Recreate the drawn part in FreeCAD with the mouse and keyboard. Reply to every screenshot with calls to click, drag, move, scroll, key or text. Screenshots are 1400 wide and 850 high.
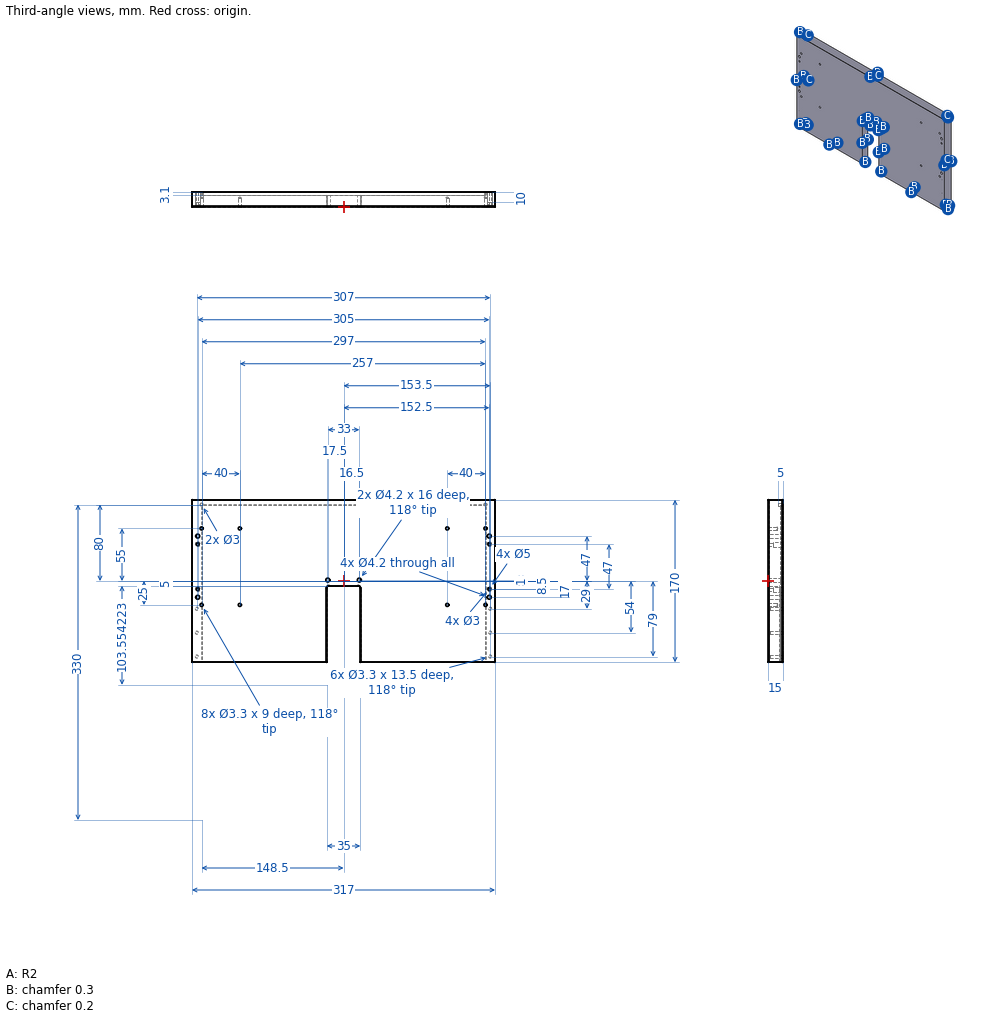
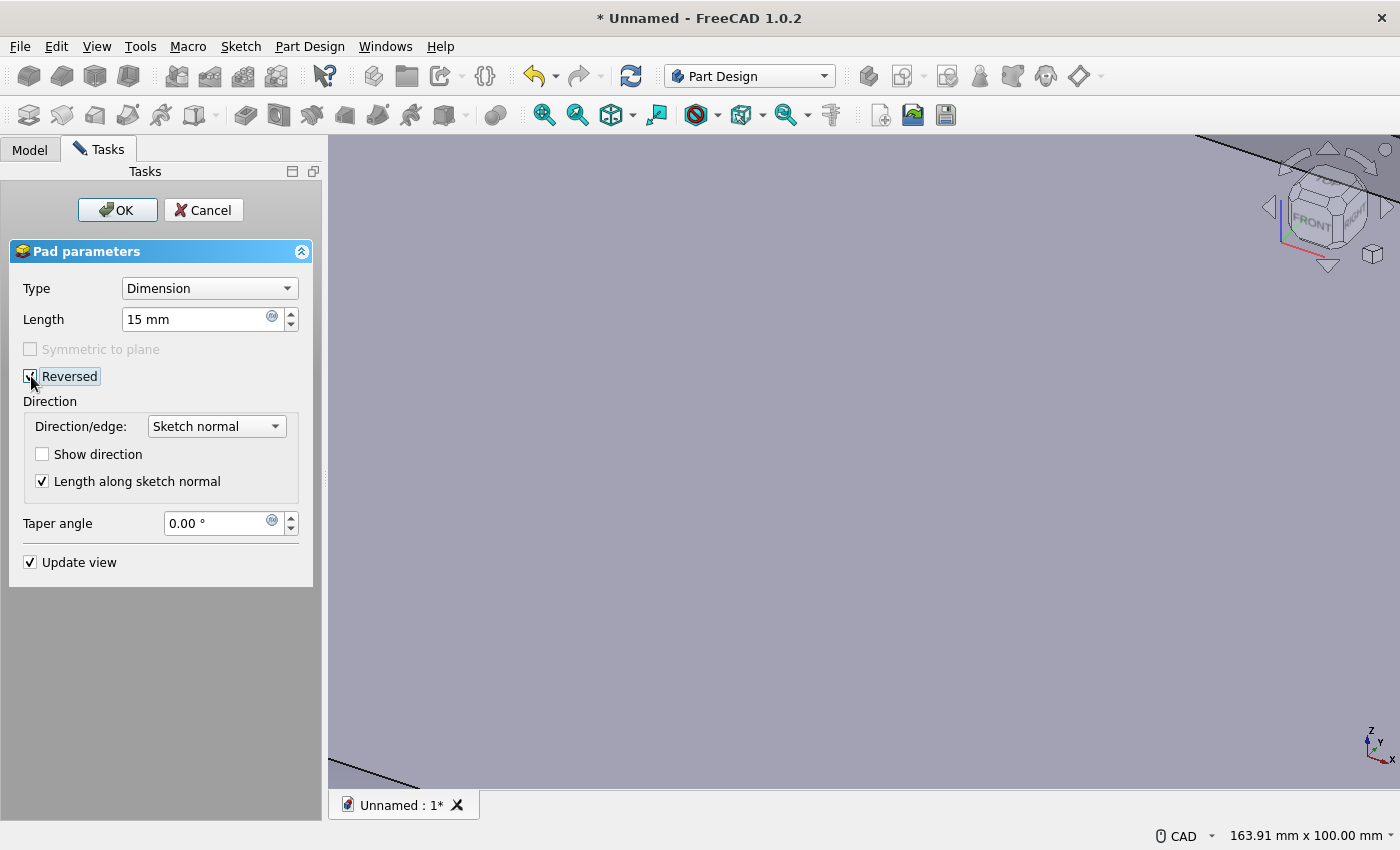
click(118, 210)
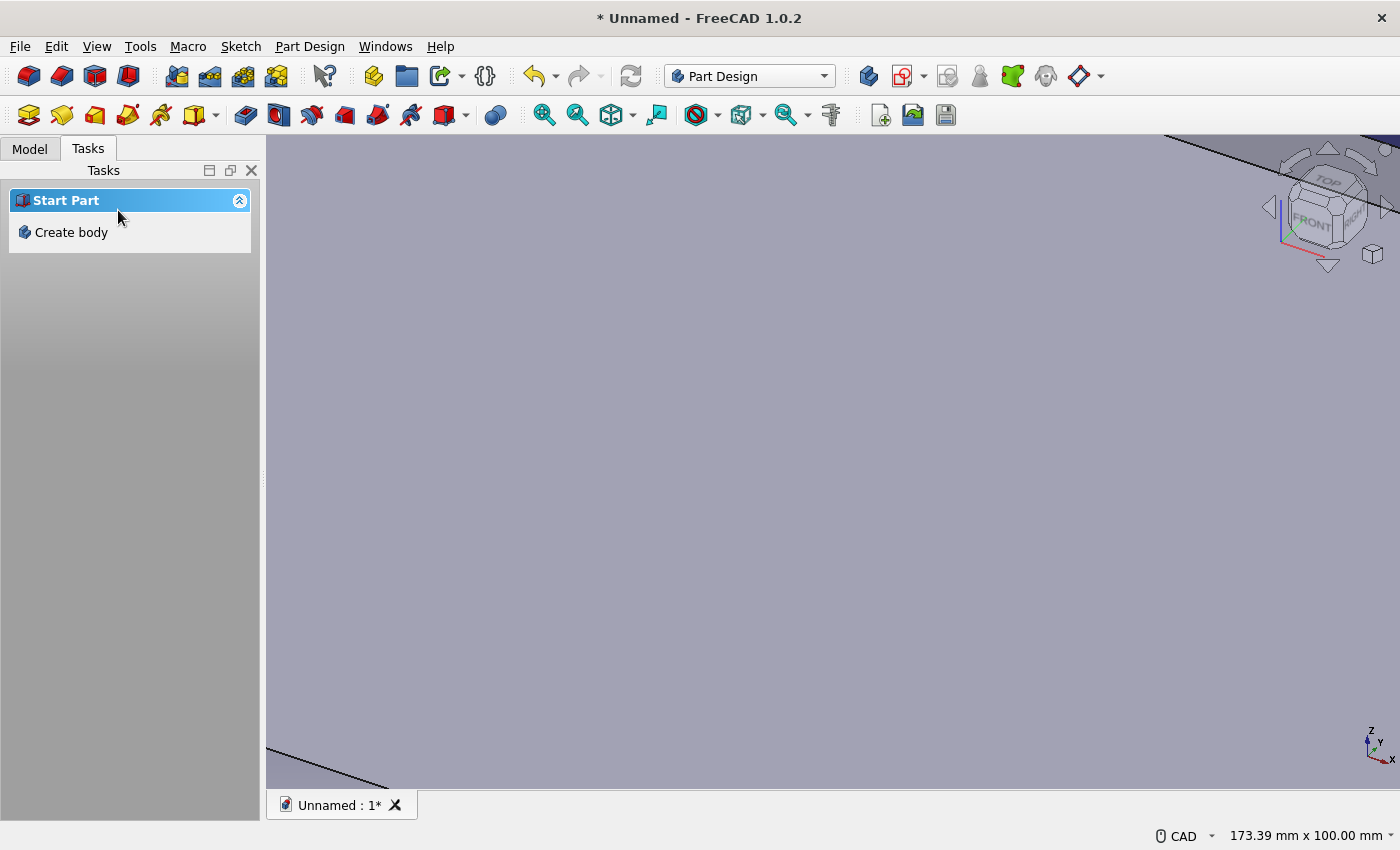
key(v)
key(f)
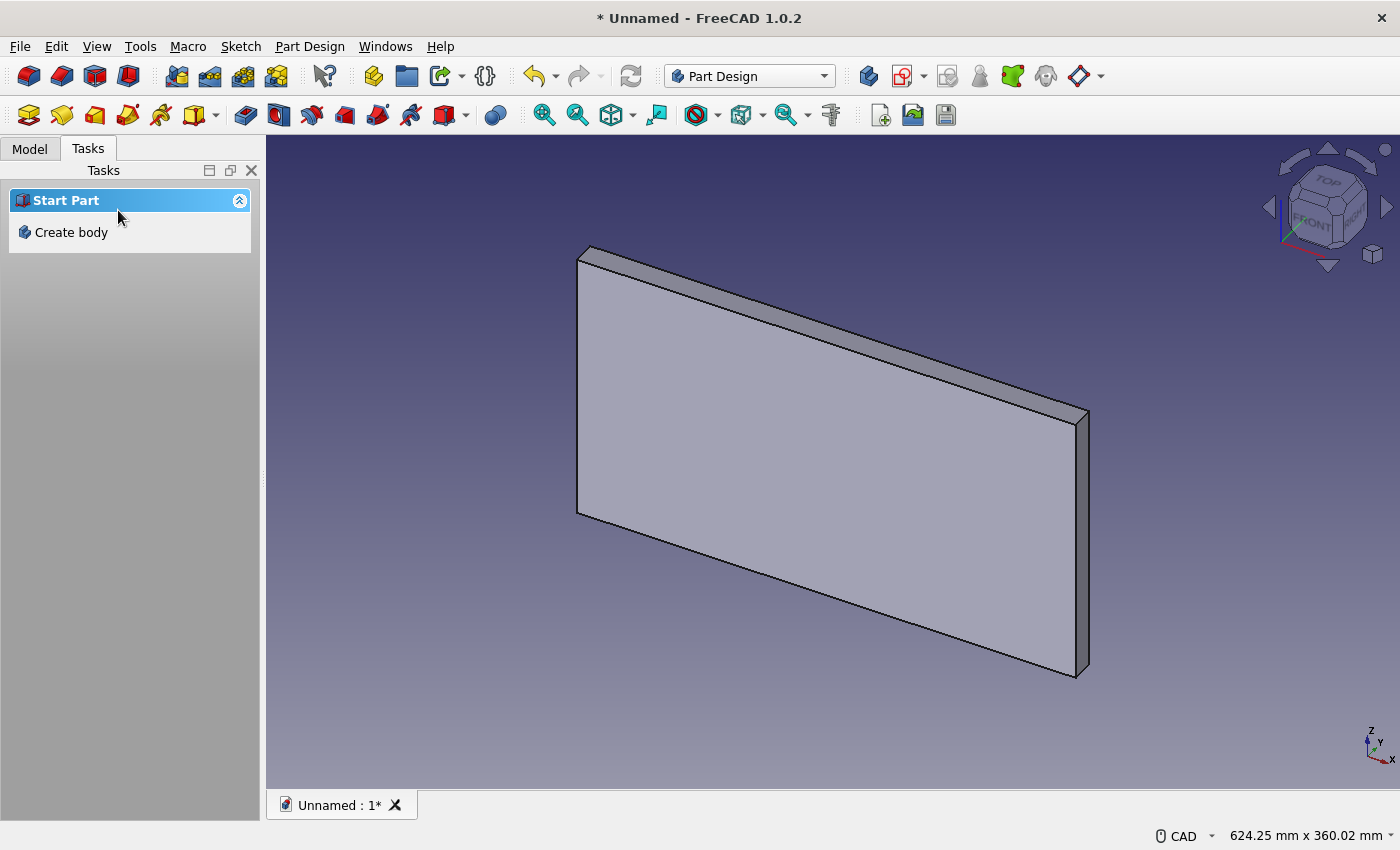
key(4)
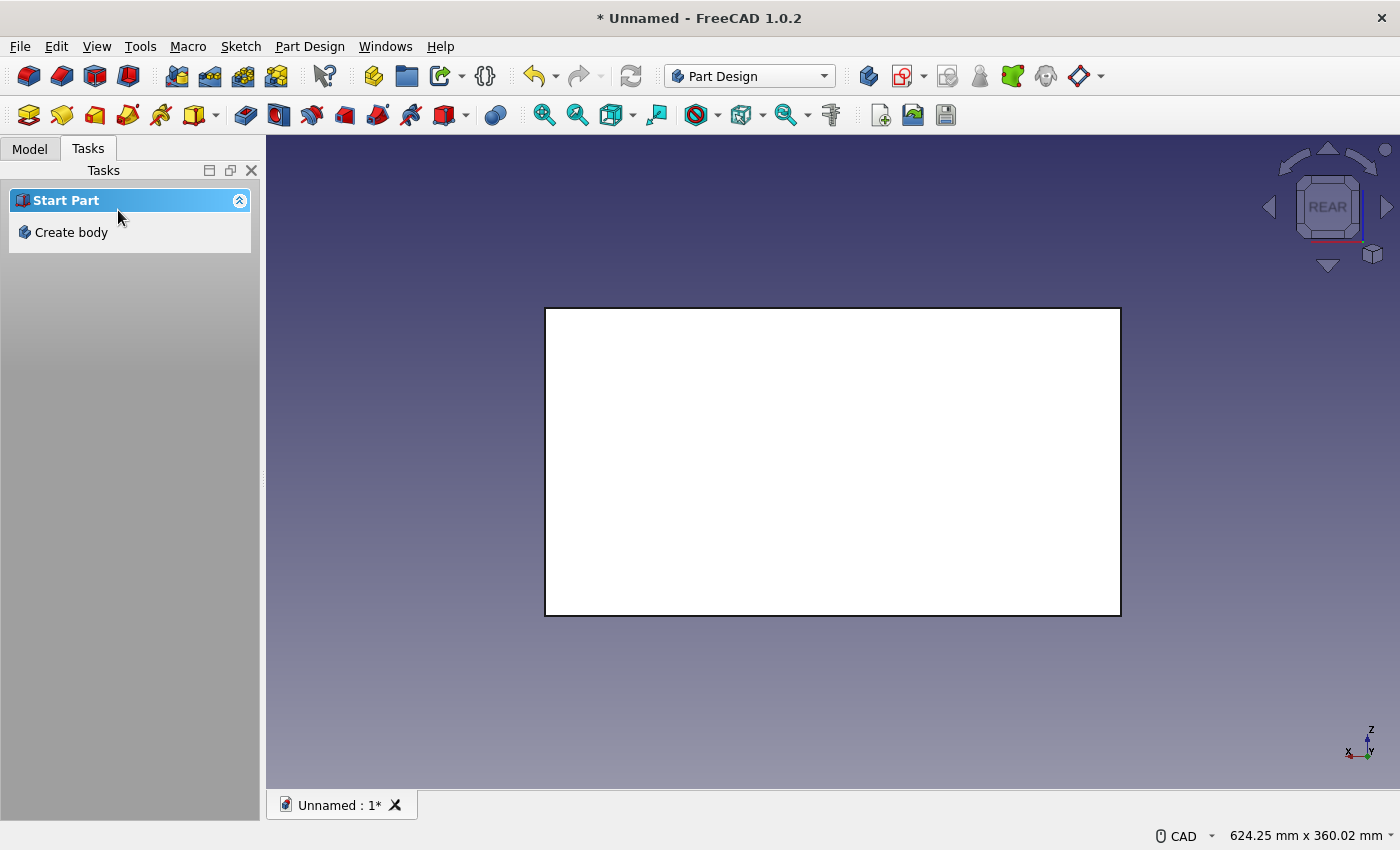
click(751, 461)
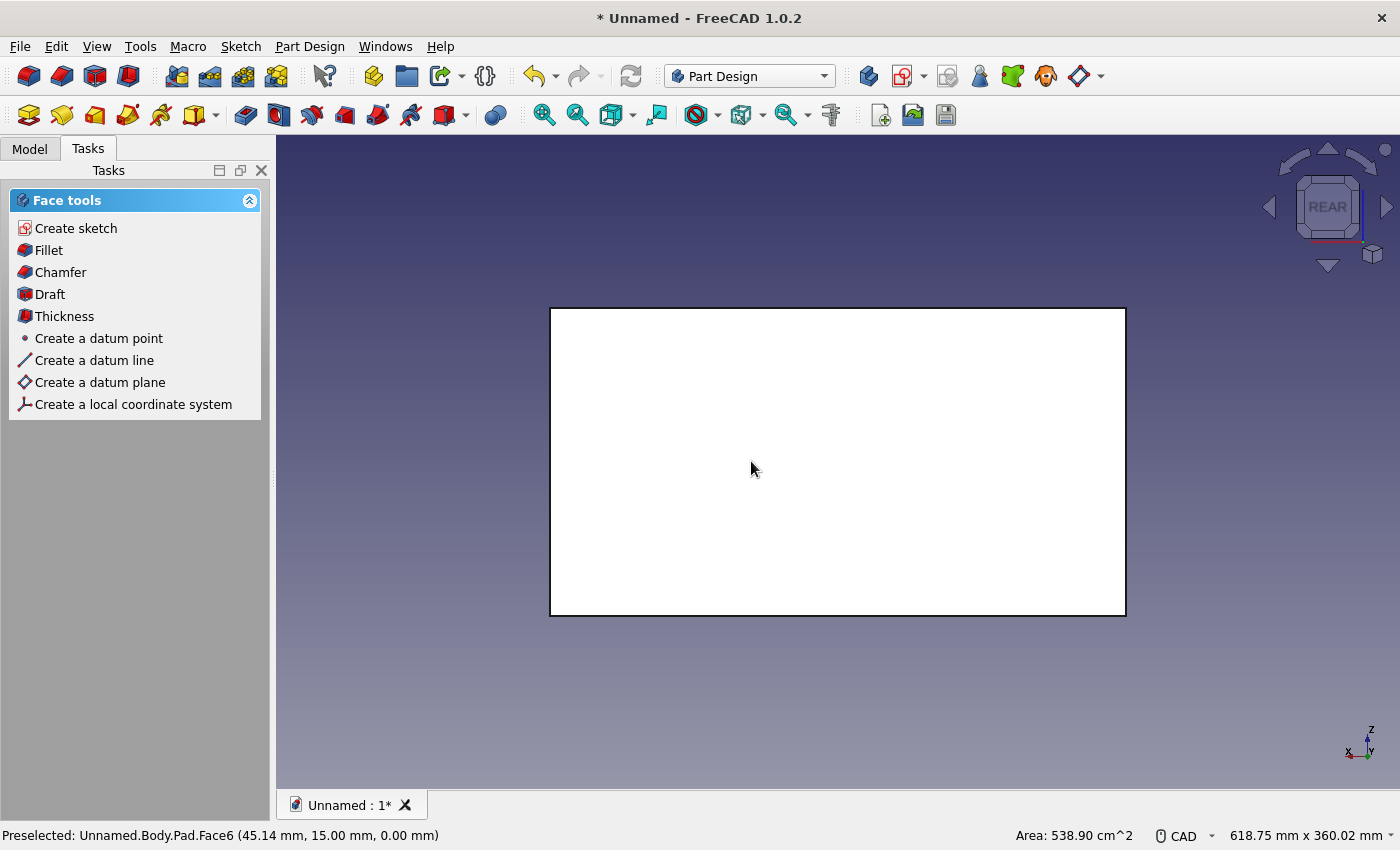
click(902, 76)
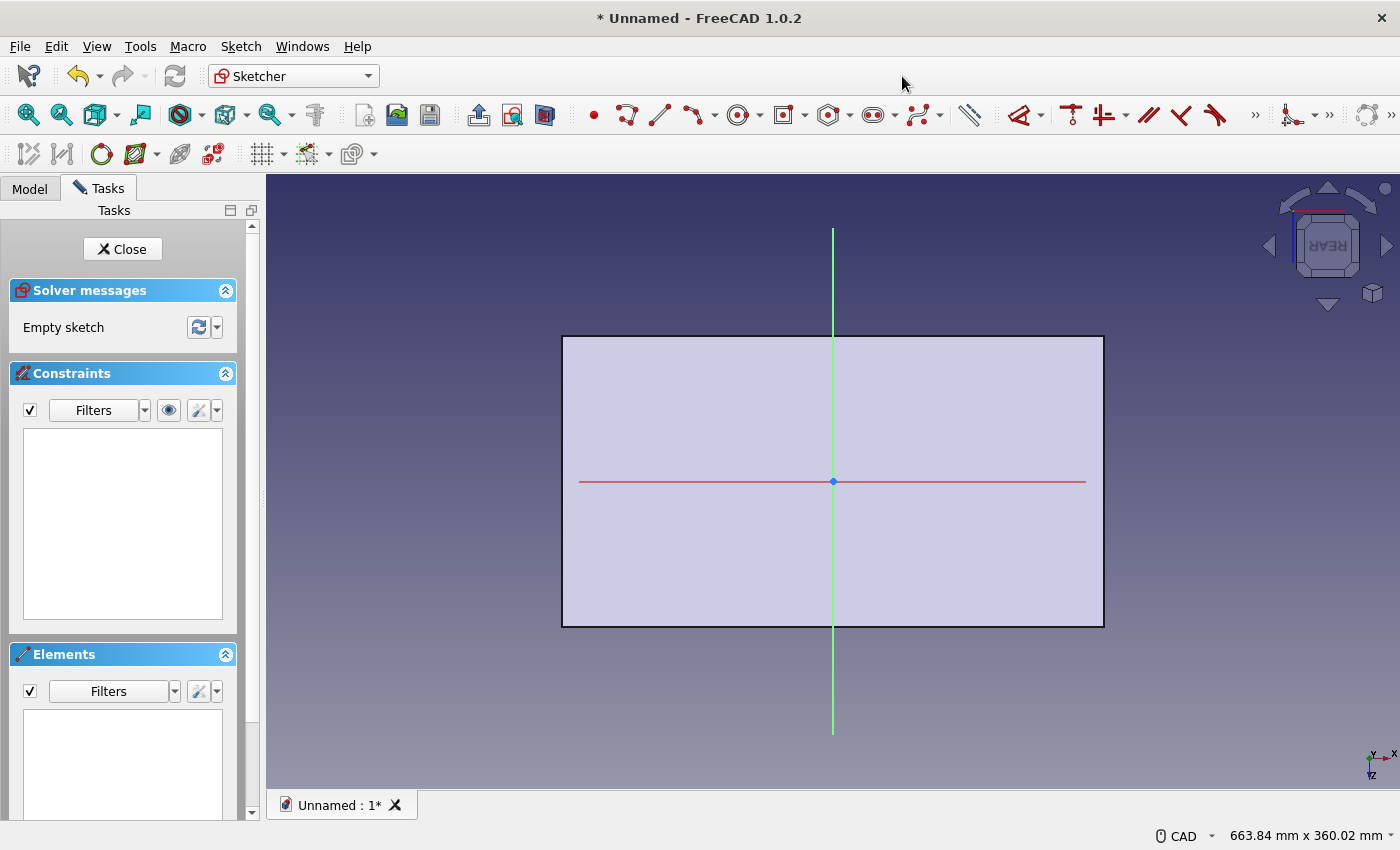
scroll(625, 761, down, 2)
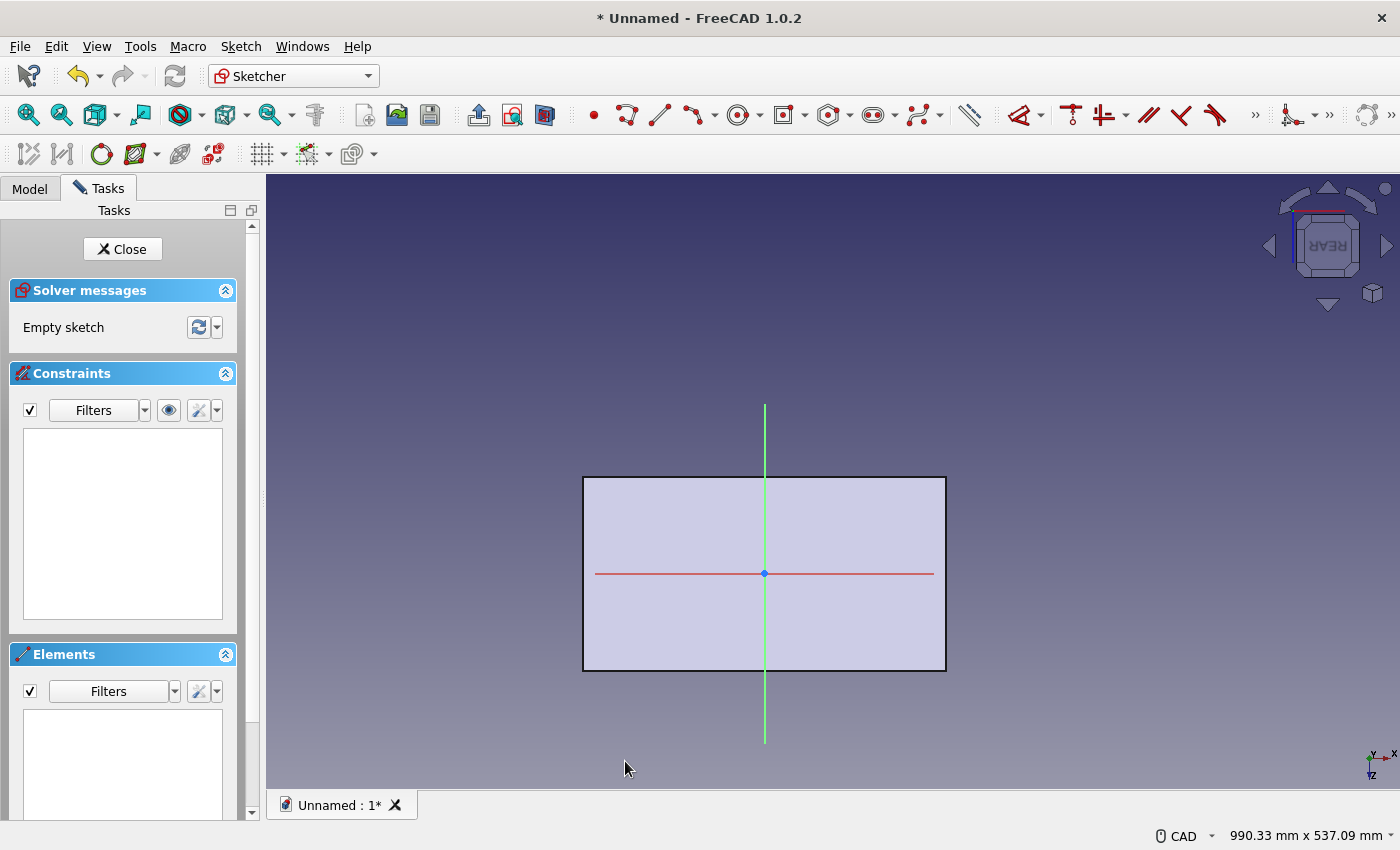
key(g)
key(r)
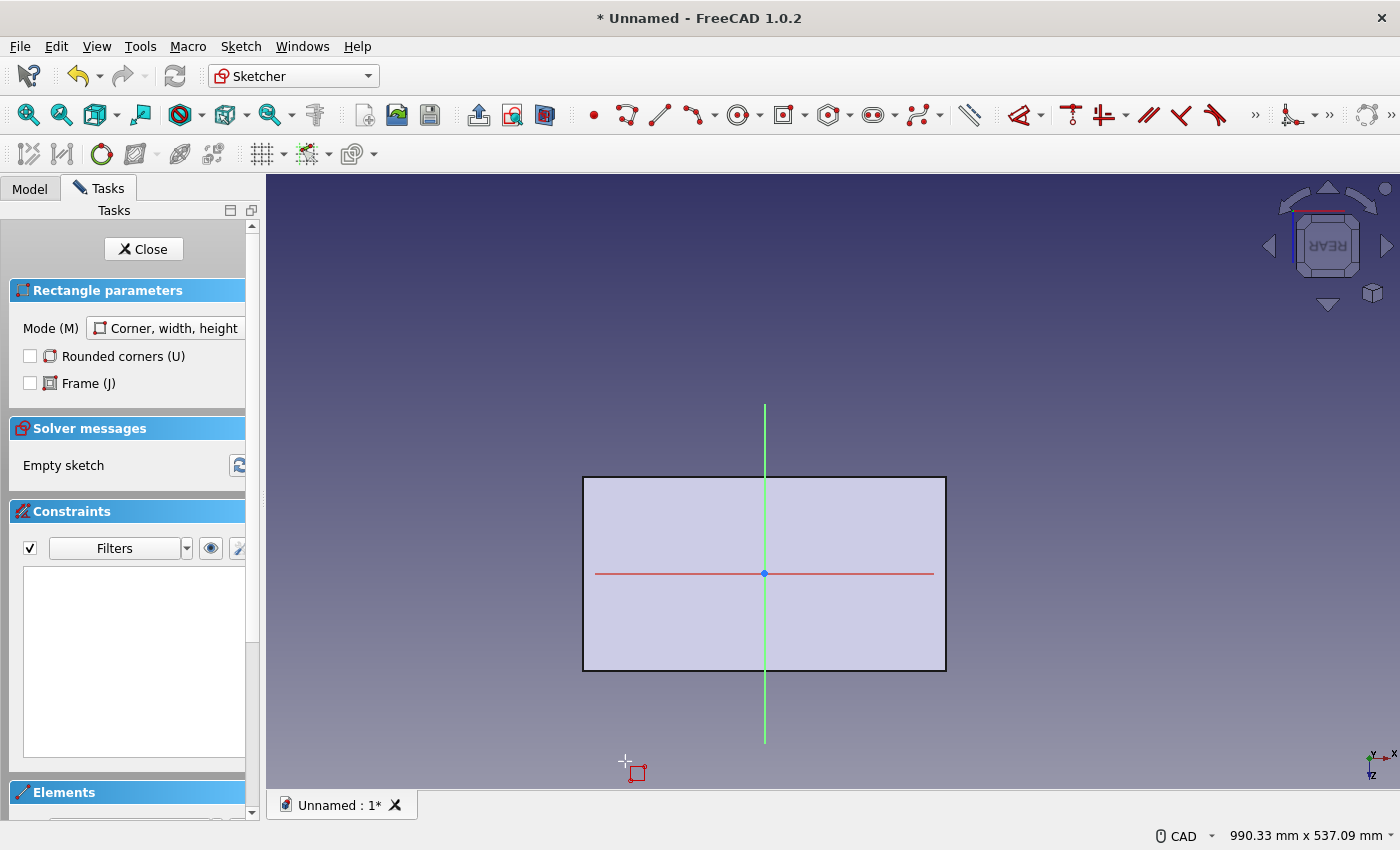
click(594, 288)
click(935, 666)
key(Escape)